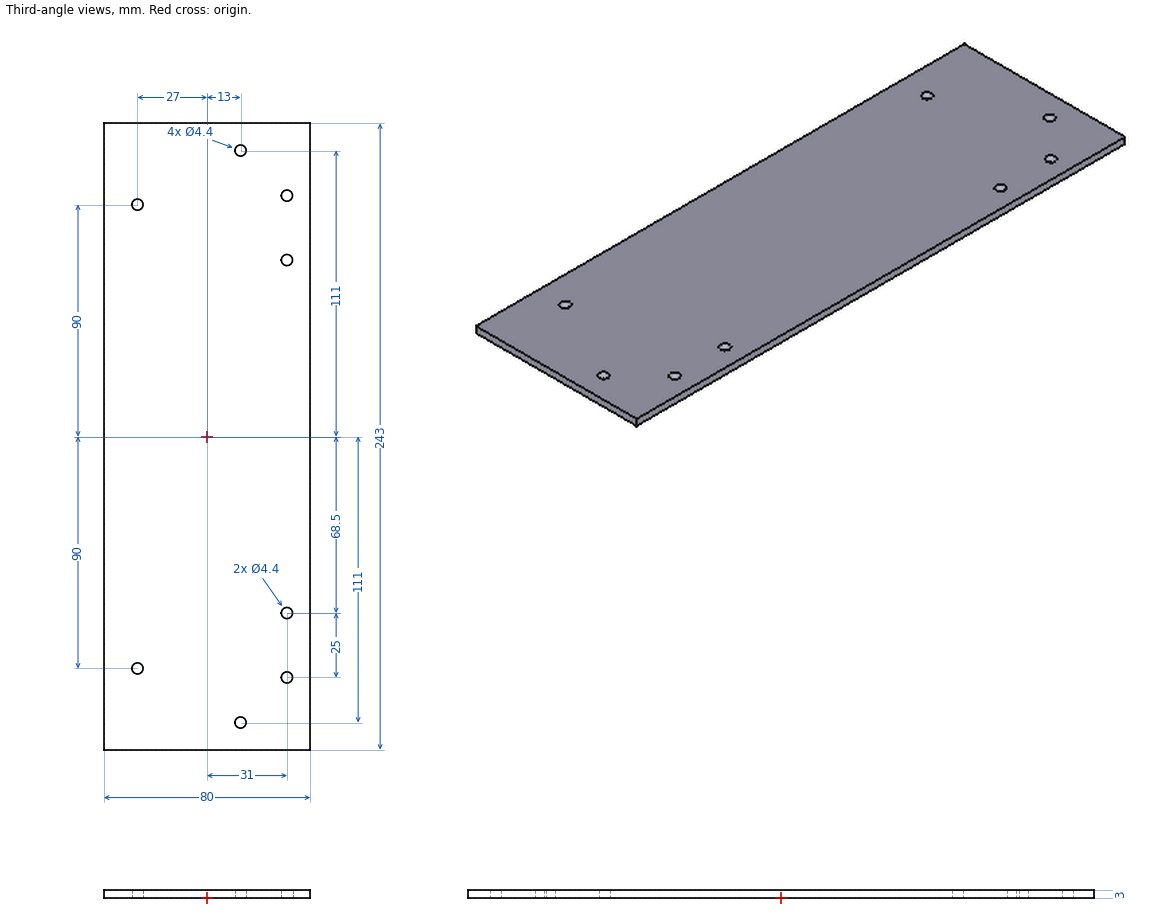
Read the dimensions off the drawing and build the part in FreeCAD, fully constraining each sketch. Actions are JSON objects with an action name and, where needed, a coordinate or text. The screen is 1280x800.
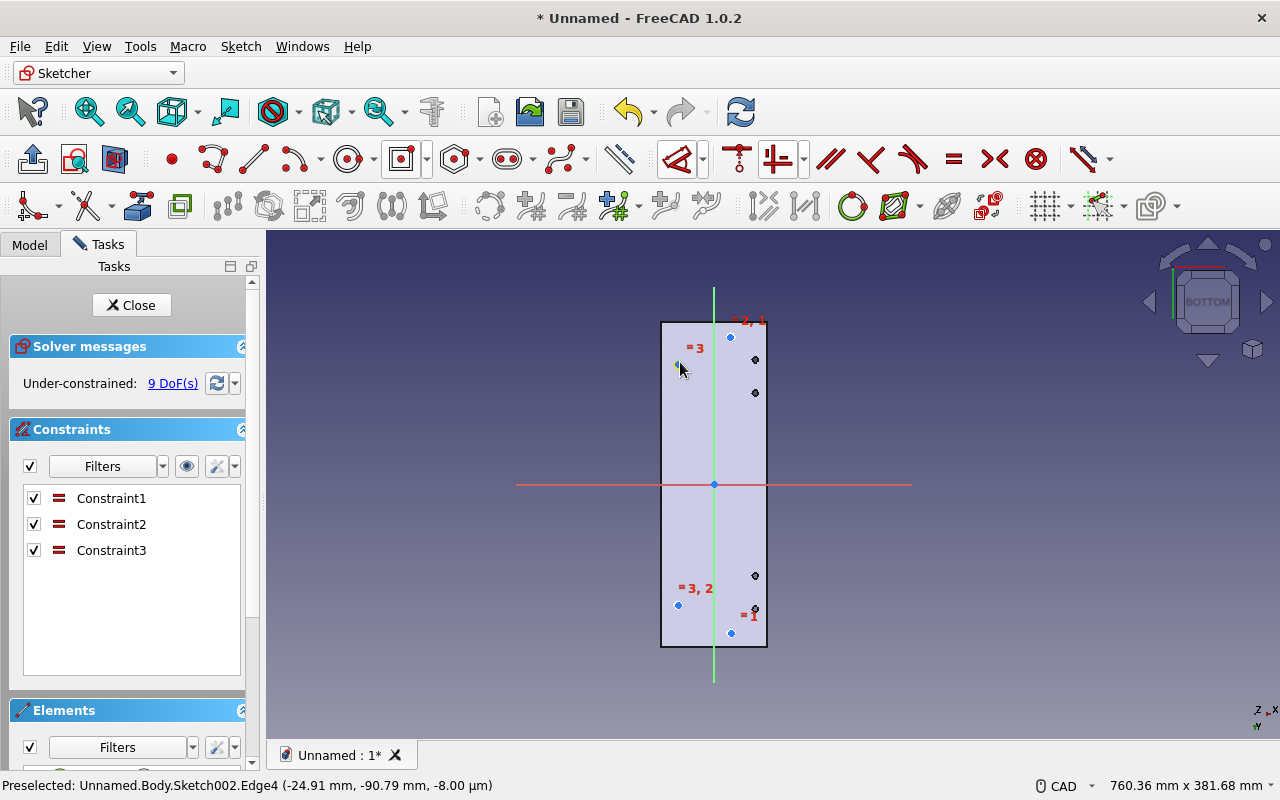
{"action": "left_click", "coordinate": [731, 633]}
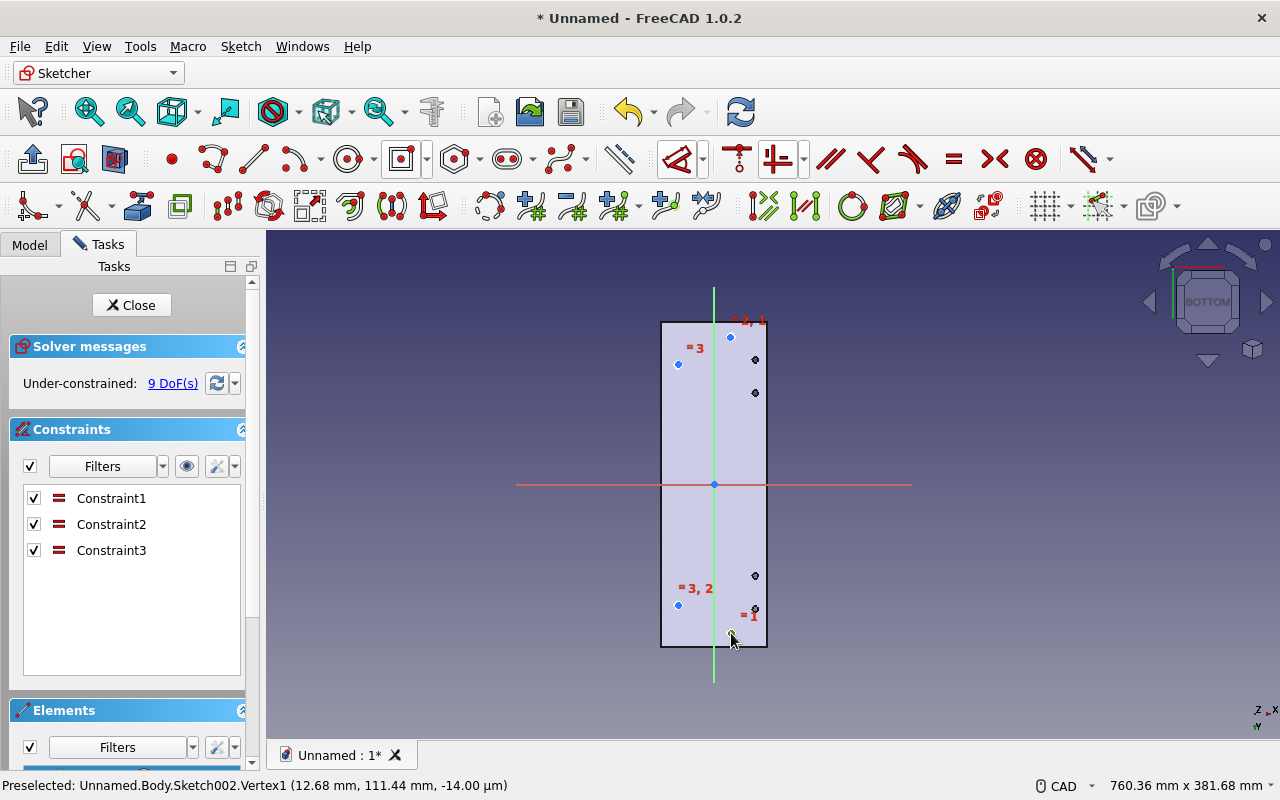
{"action": "left_click", "coordinate": [731, 337]}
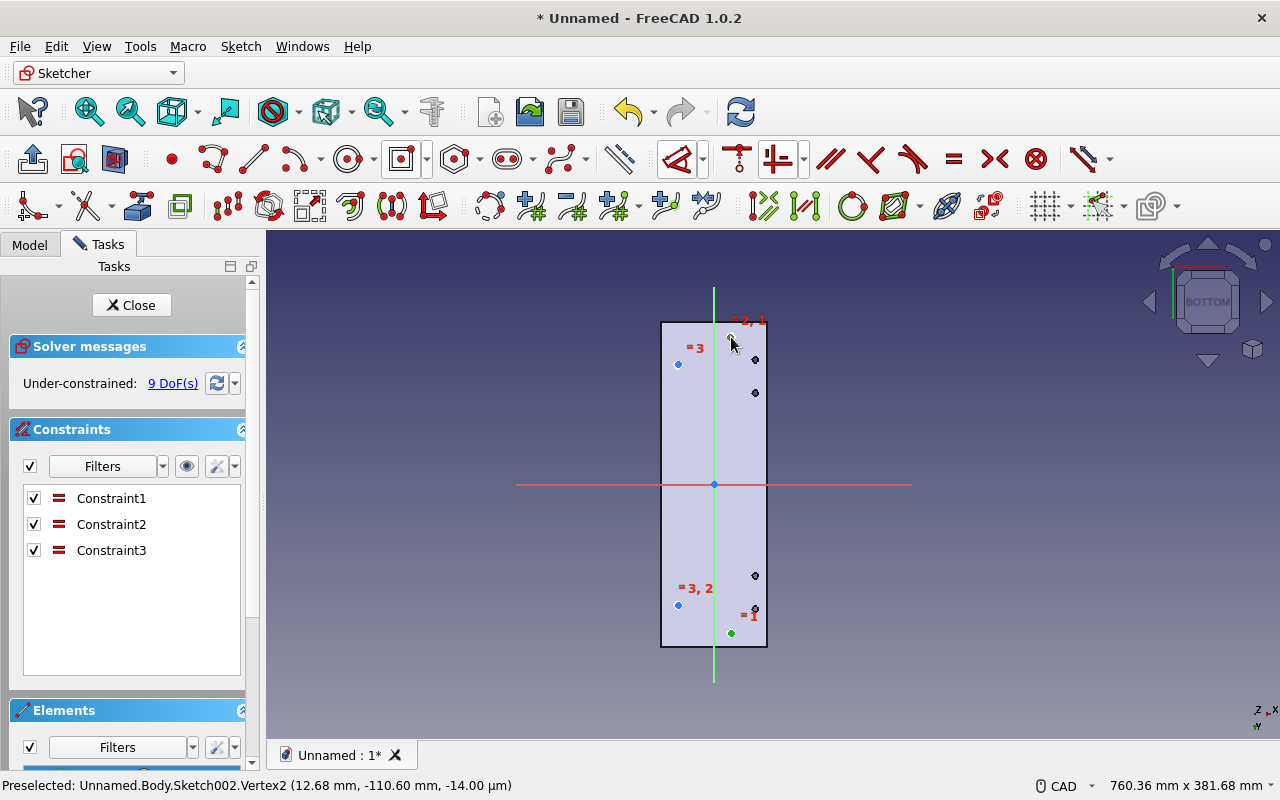
{"action": "left_click", "coordinate": [804, 160]}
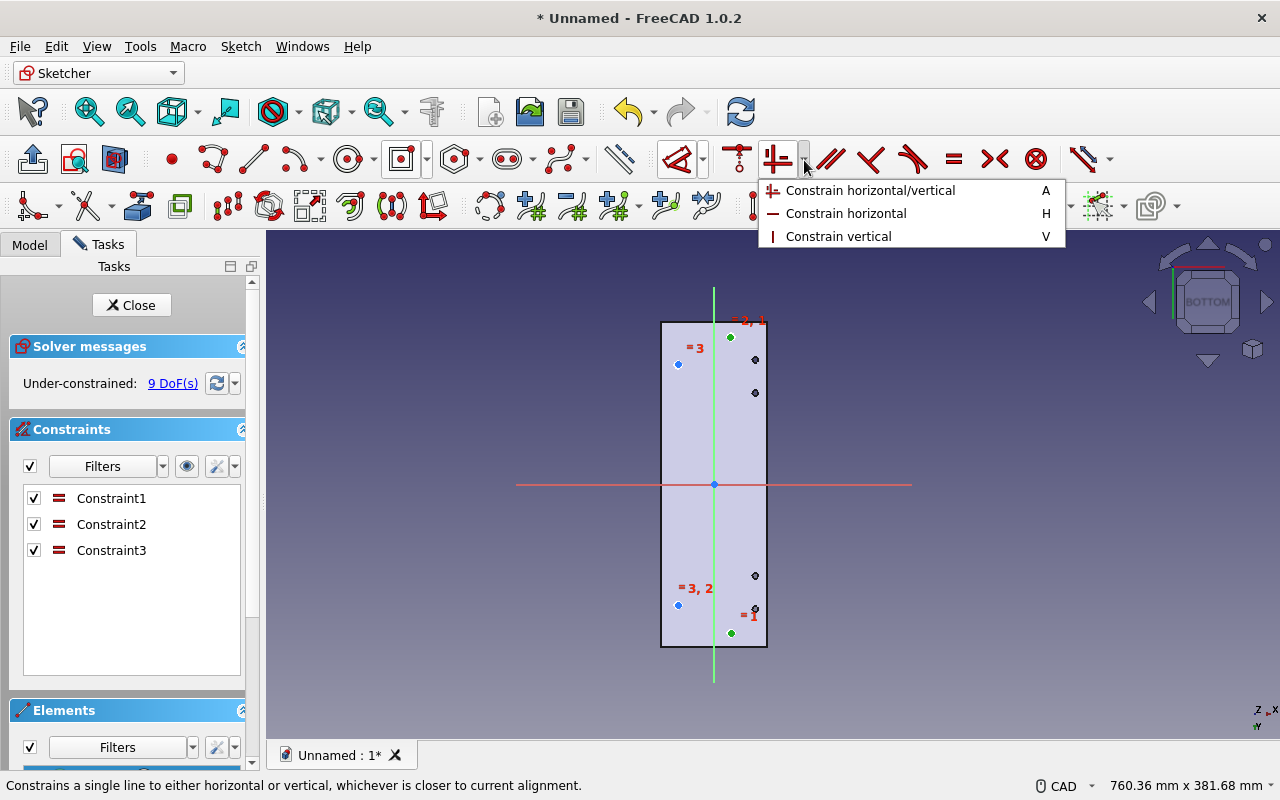
{"action": "left_click", "coordinate": [912, 236]}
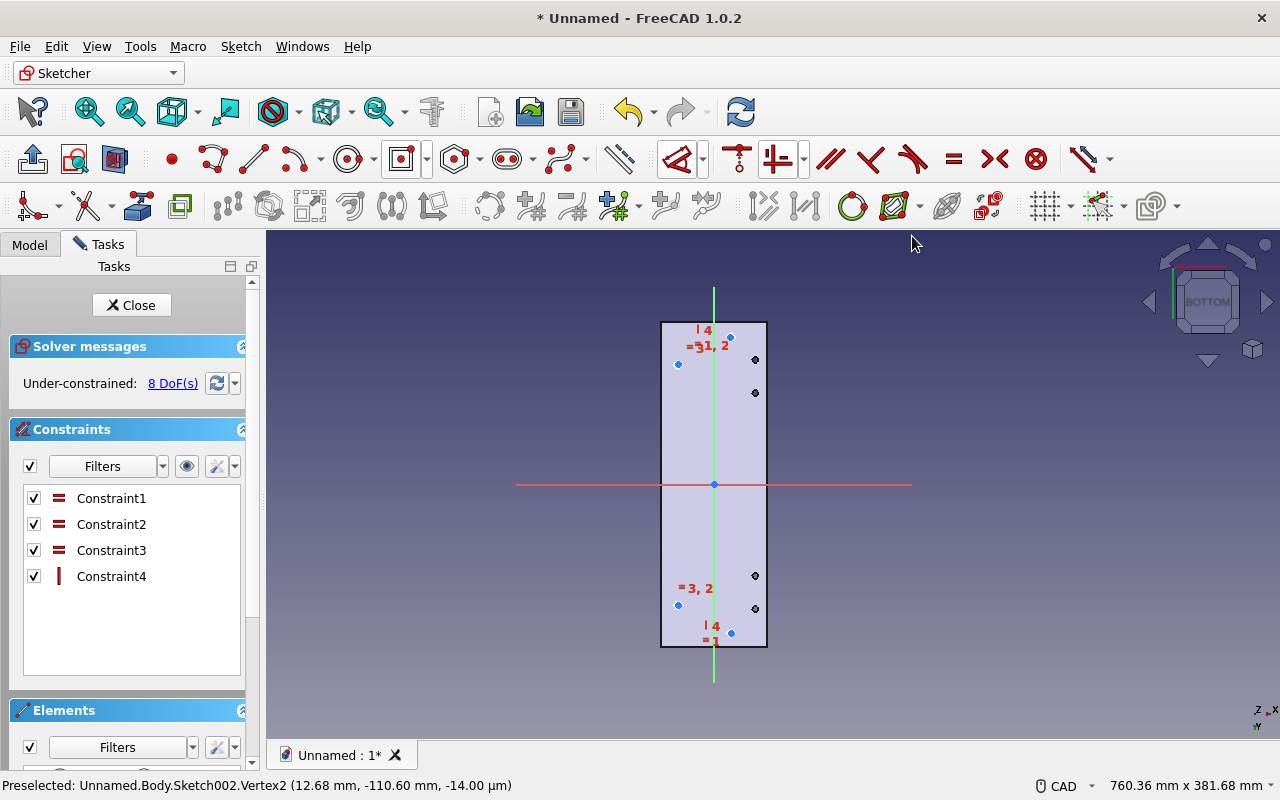
{"action": "left_click", "coordinate": [678, 605]}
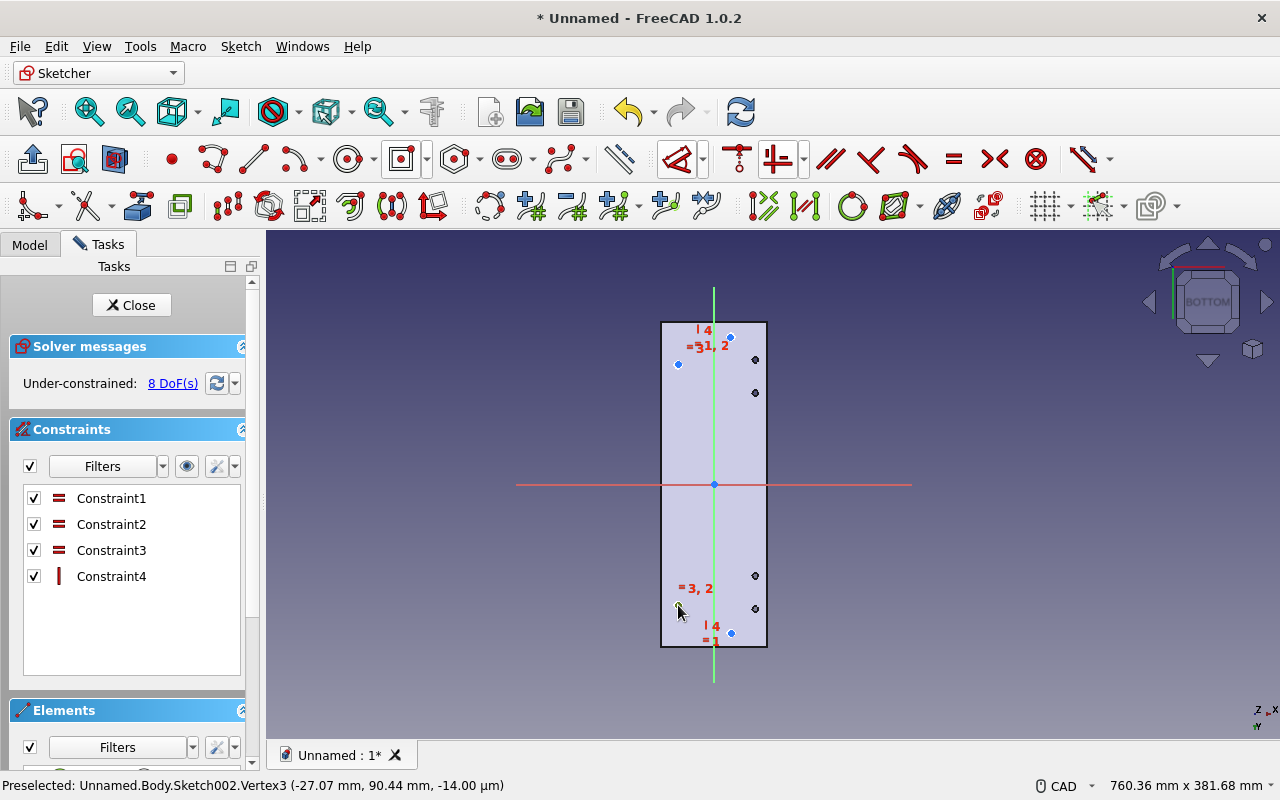
{"action": "left_click", "coordinate": [678, 365]}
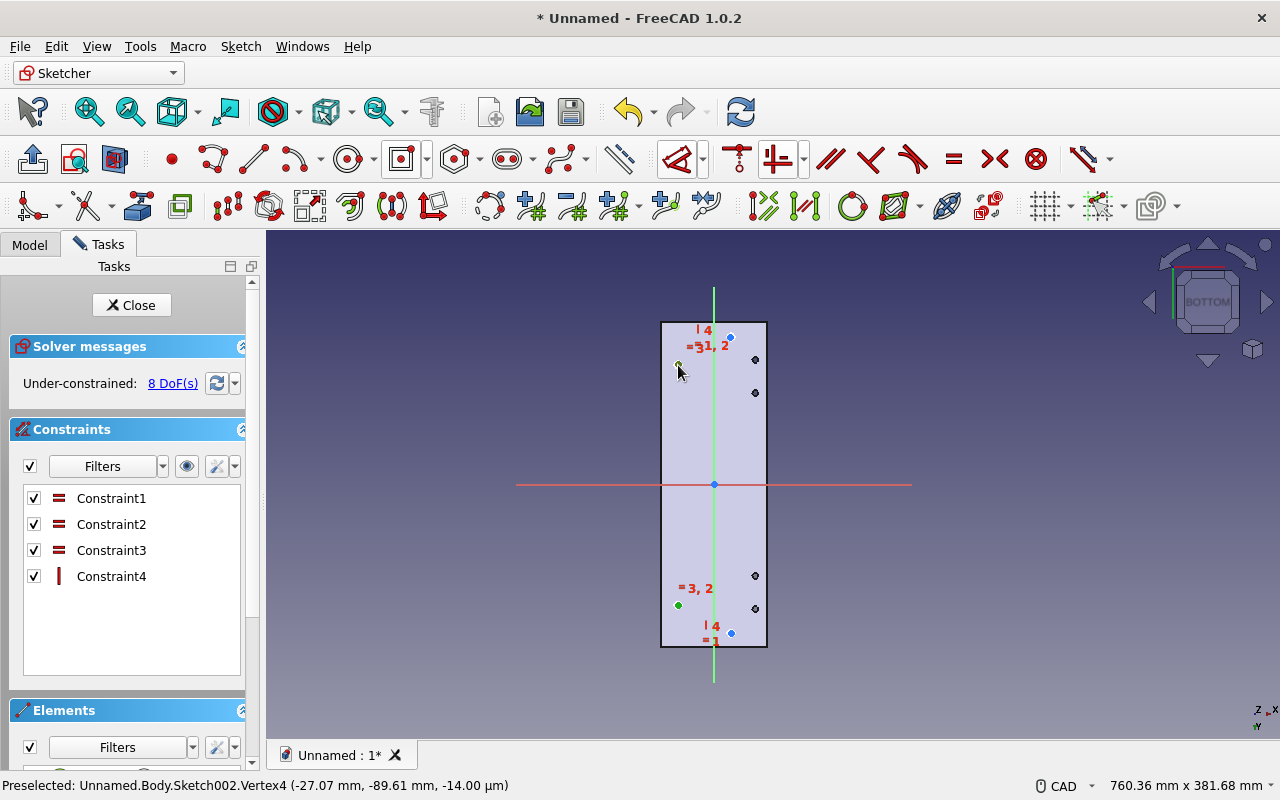
{"action": "key", "text": "v"}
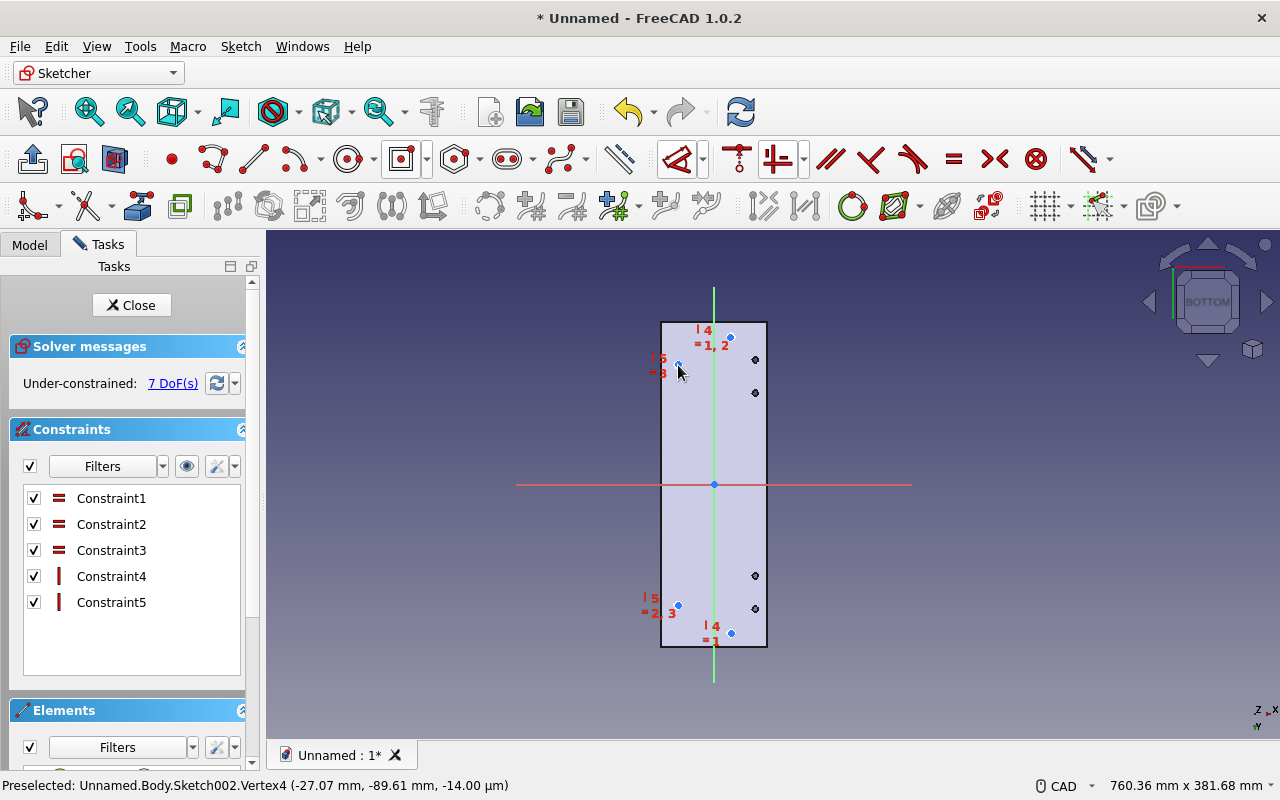
{"action": "scroll", "coordinate": [728, 631], "scroll_direction": "up", "scroll_amount": 10}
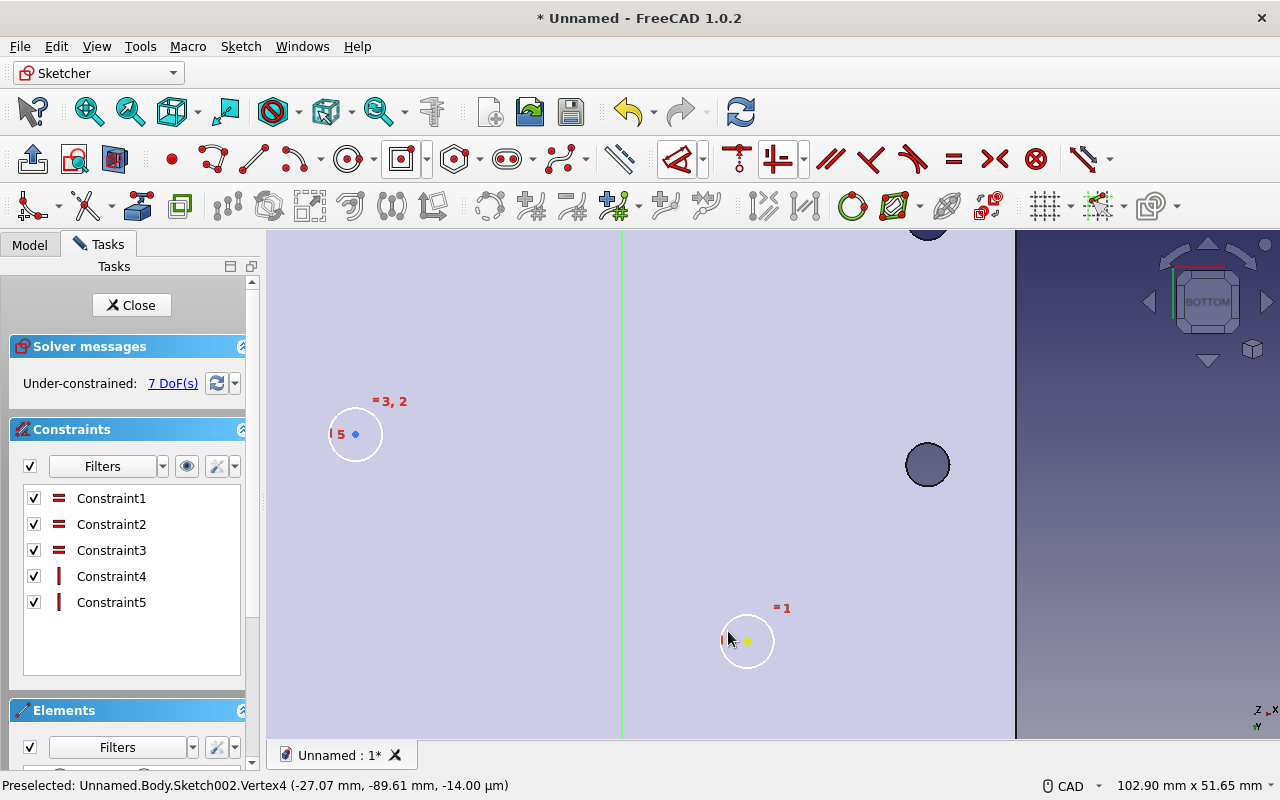
{"action": "left_click", "coordinate": [728, 623]}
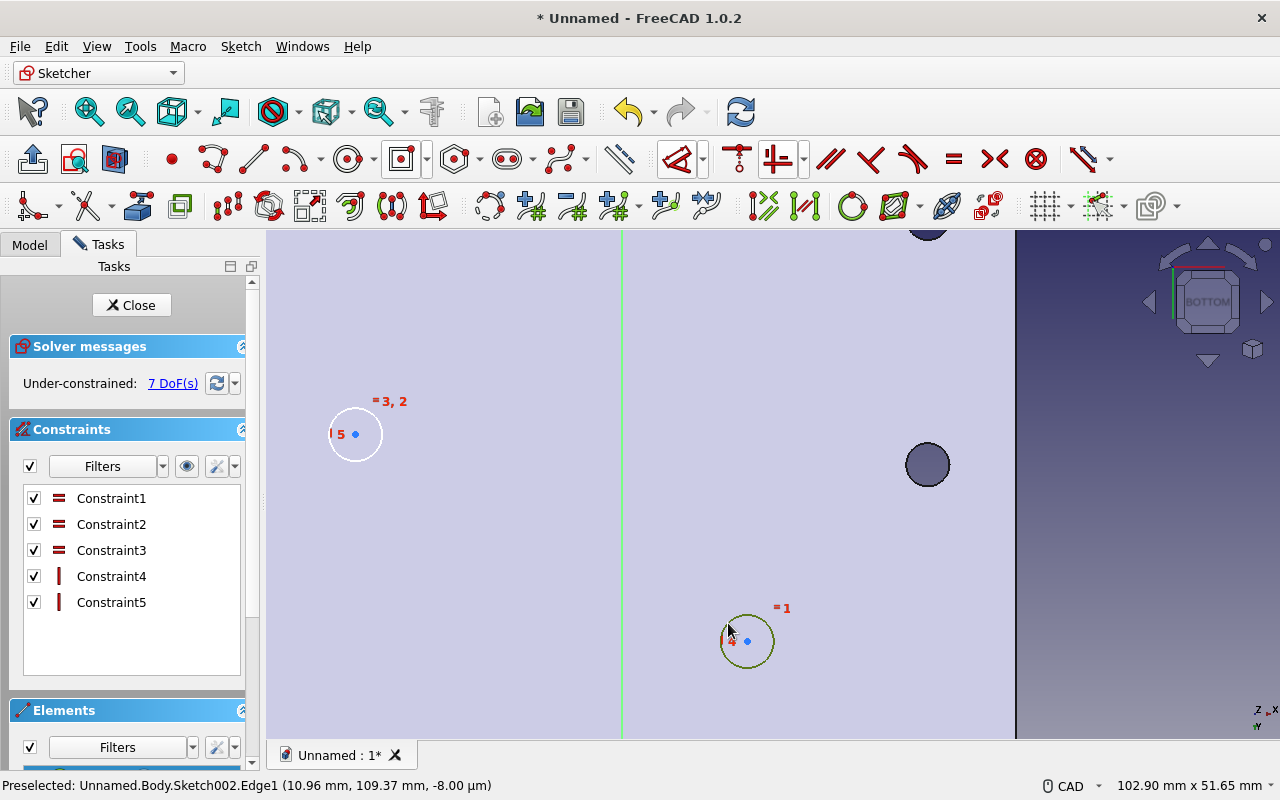
{"action": "left_click", "coordinate": [702, 160]}